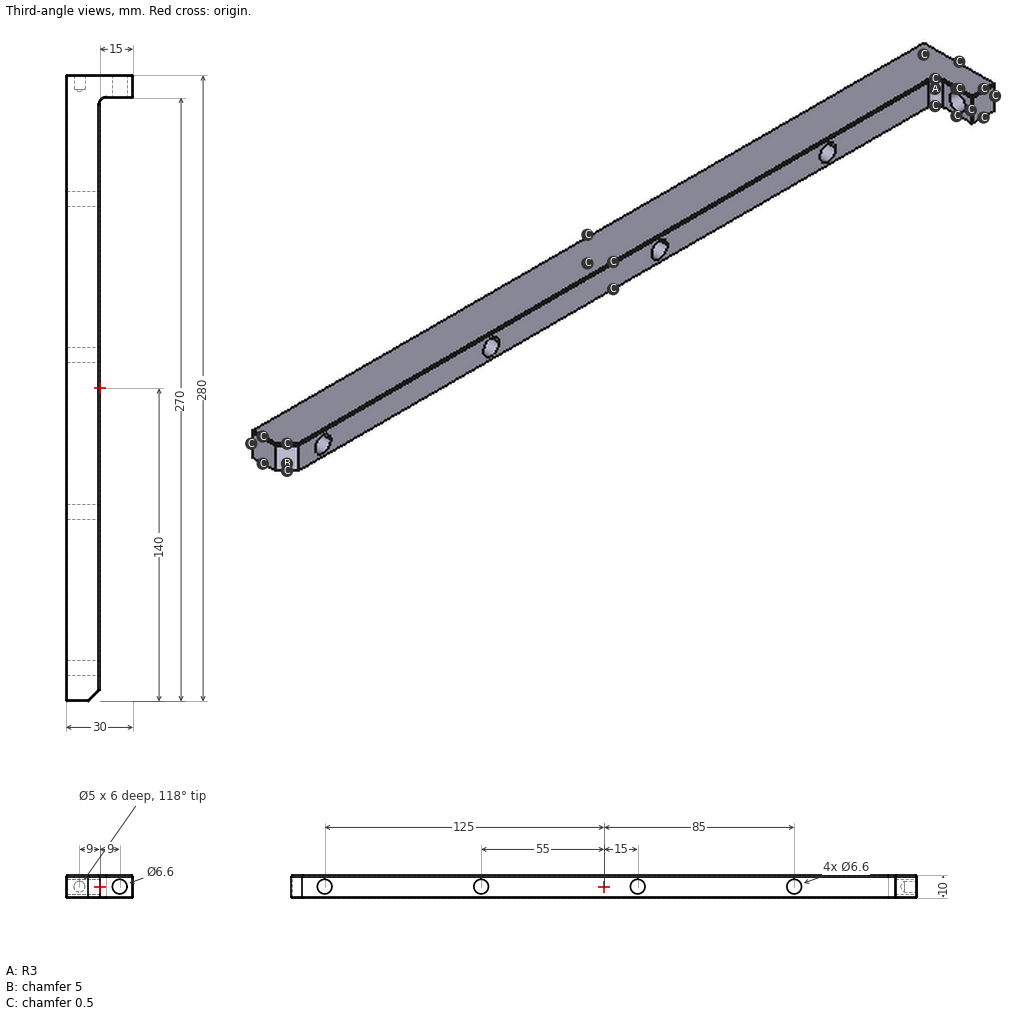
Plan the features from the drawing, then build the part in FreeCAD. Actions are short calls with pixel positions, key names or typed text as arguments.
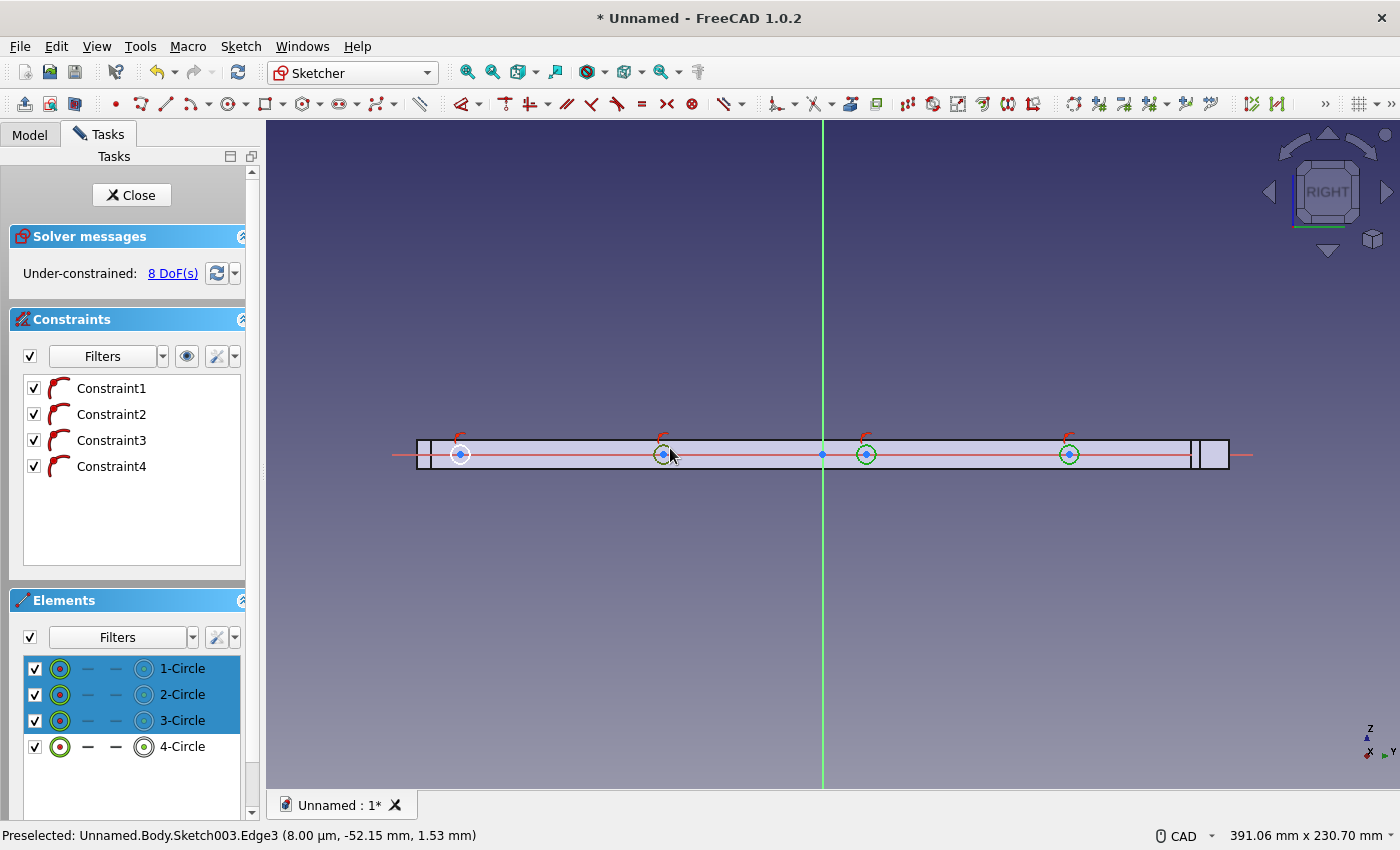
scroll(467, 448, up, 4)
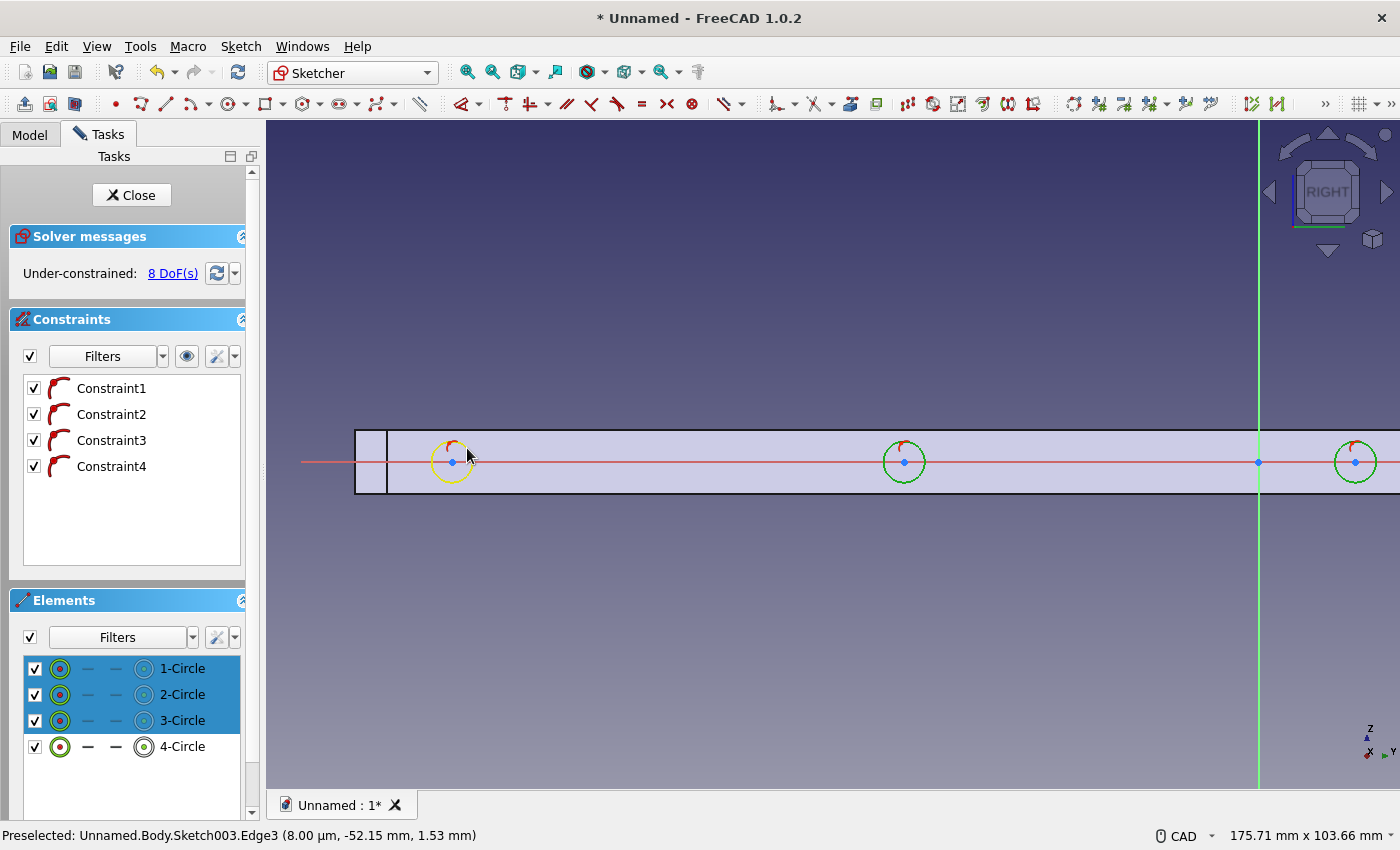
click(467, 447)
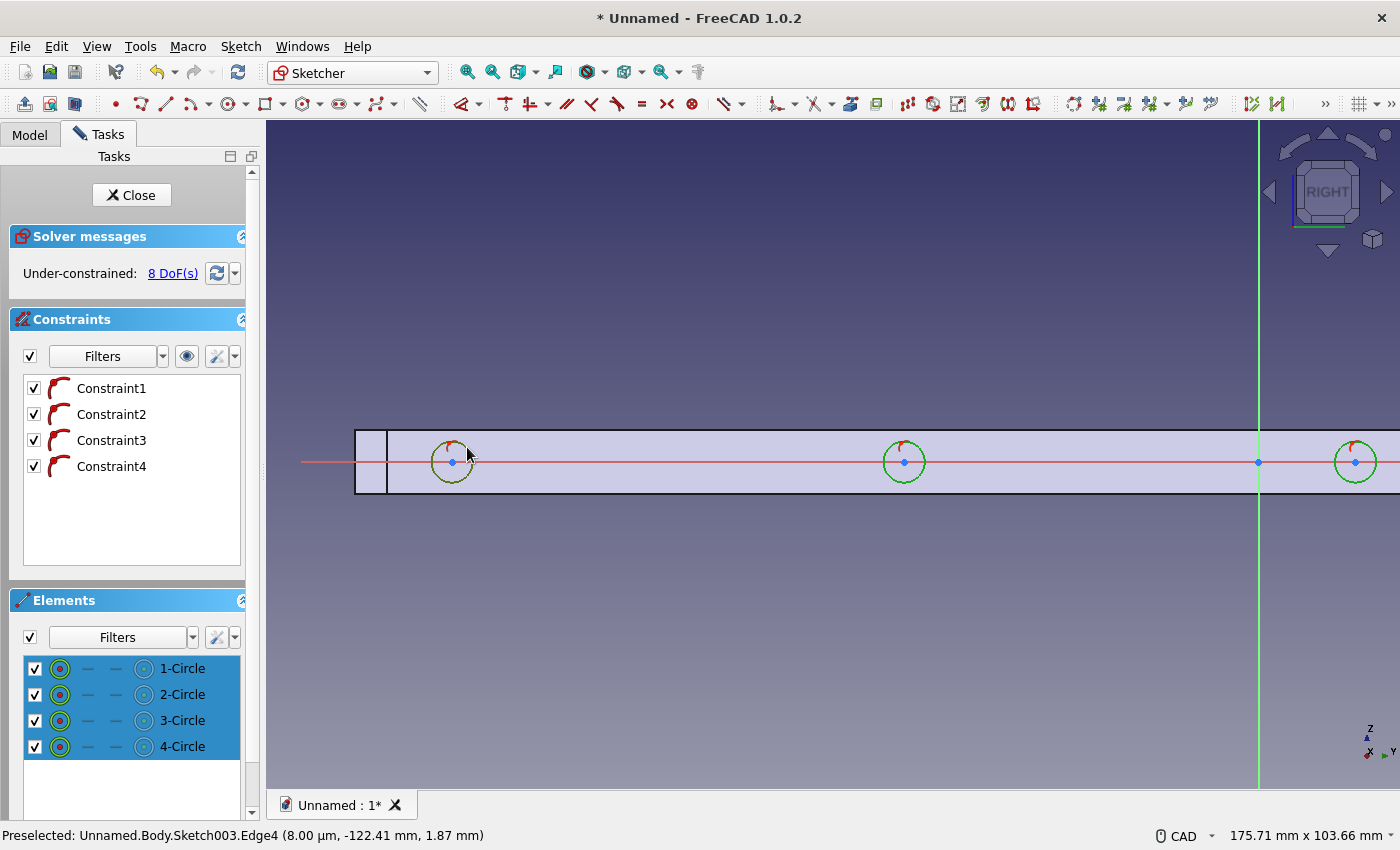
key(e)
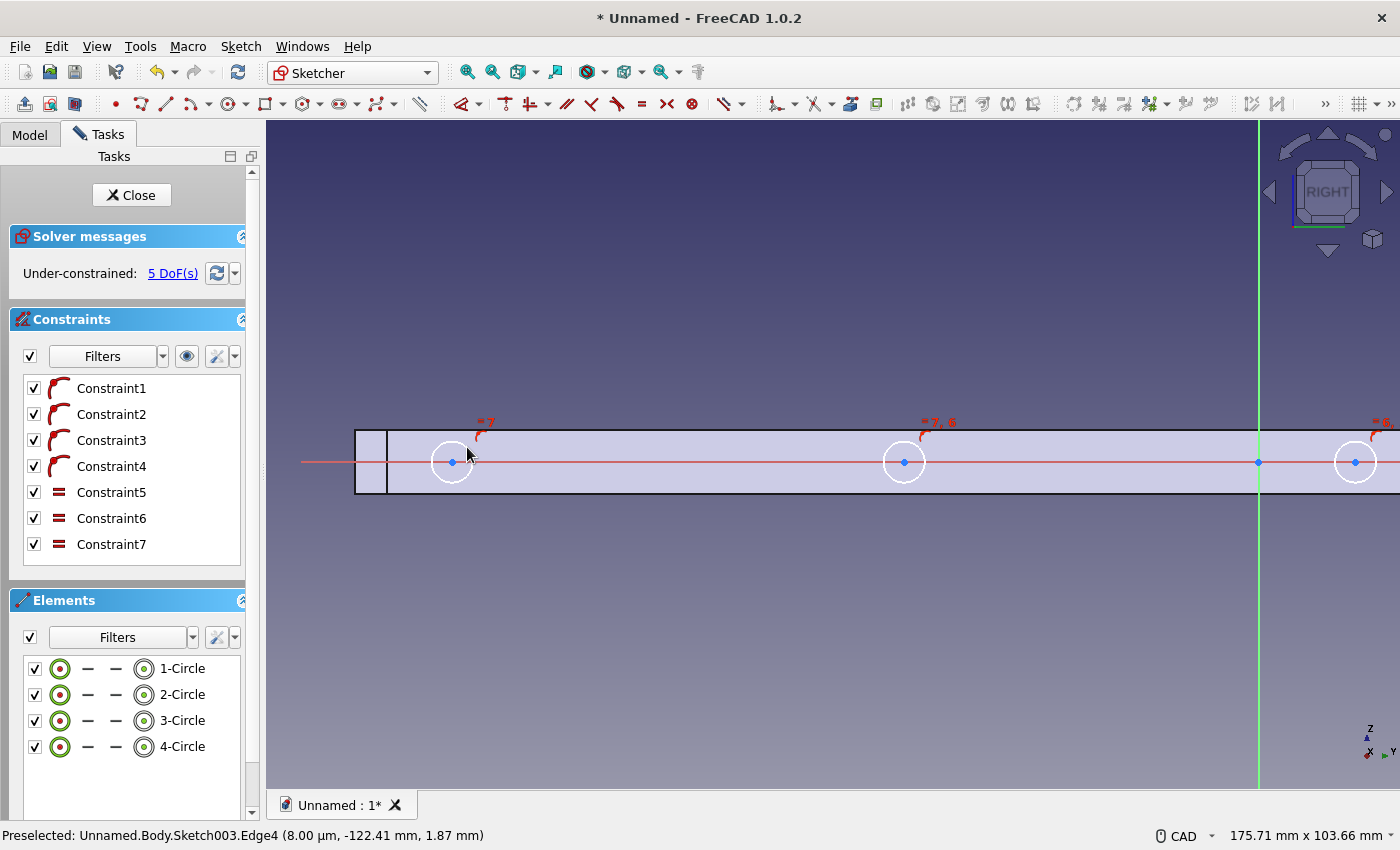
key(d)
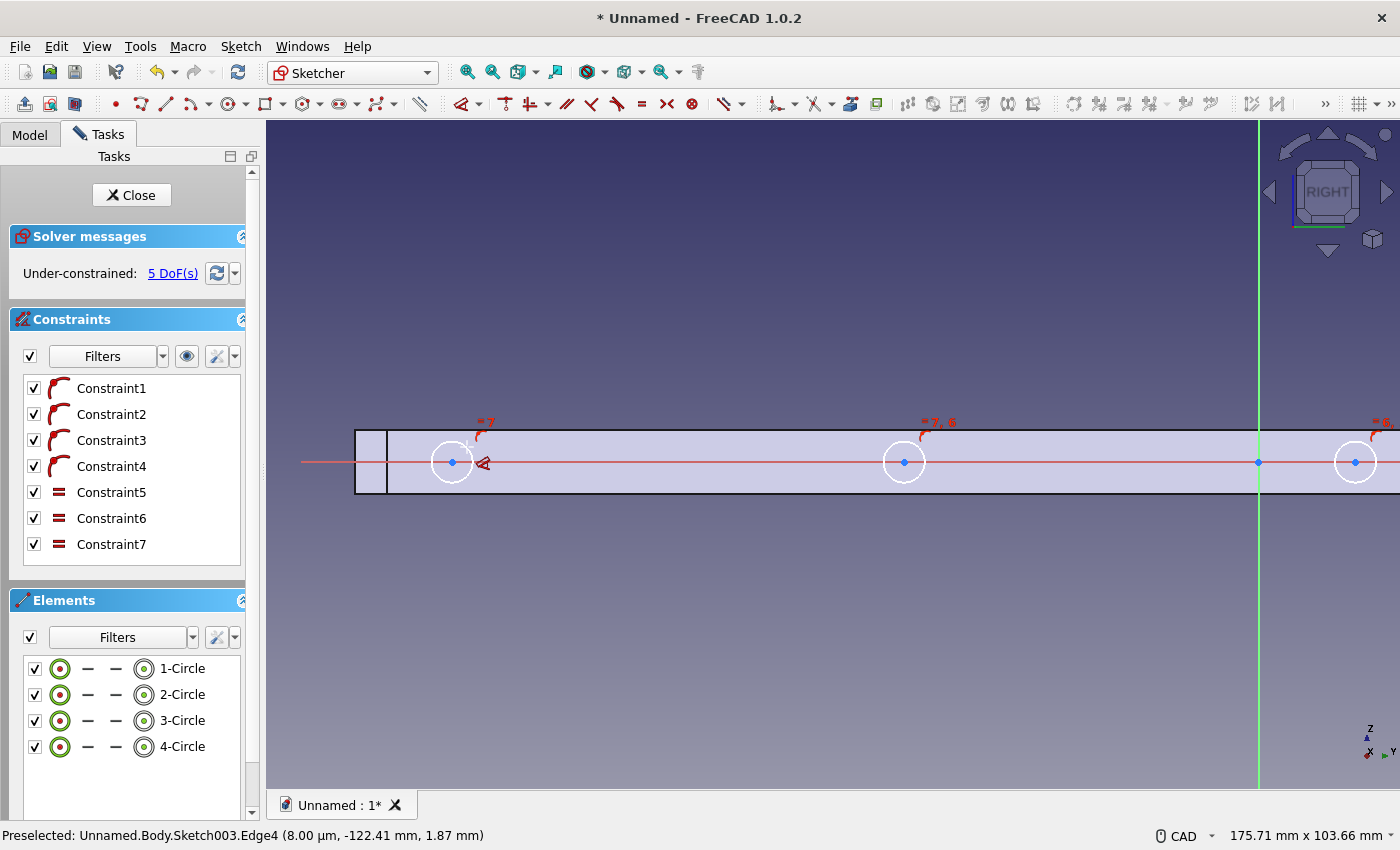
scroll(467, 448, down, 4)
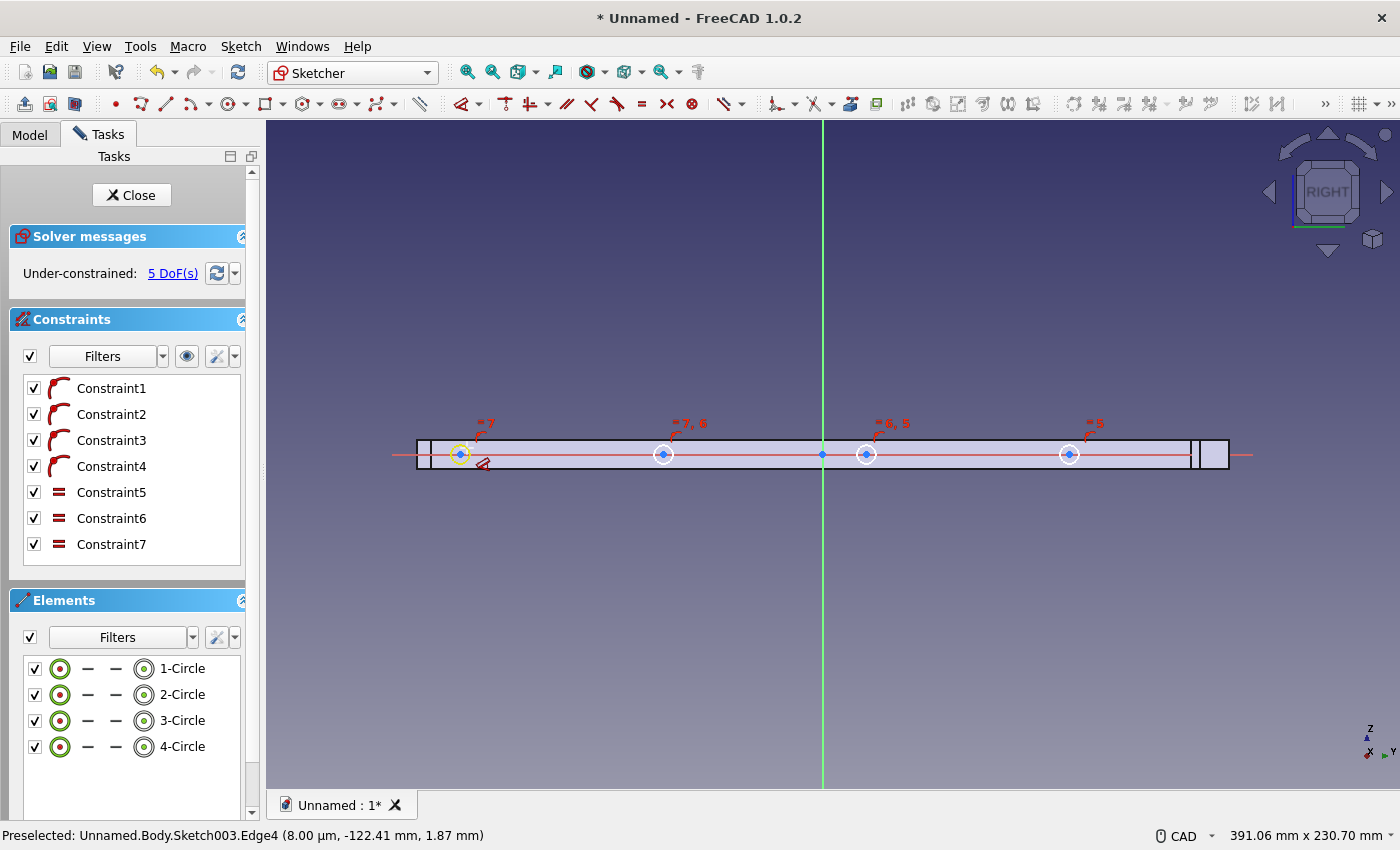
scroll(1076, 448, up, 4)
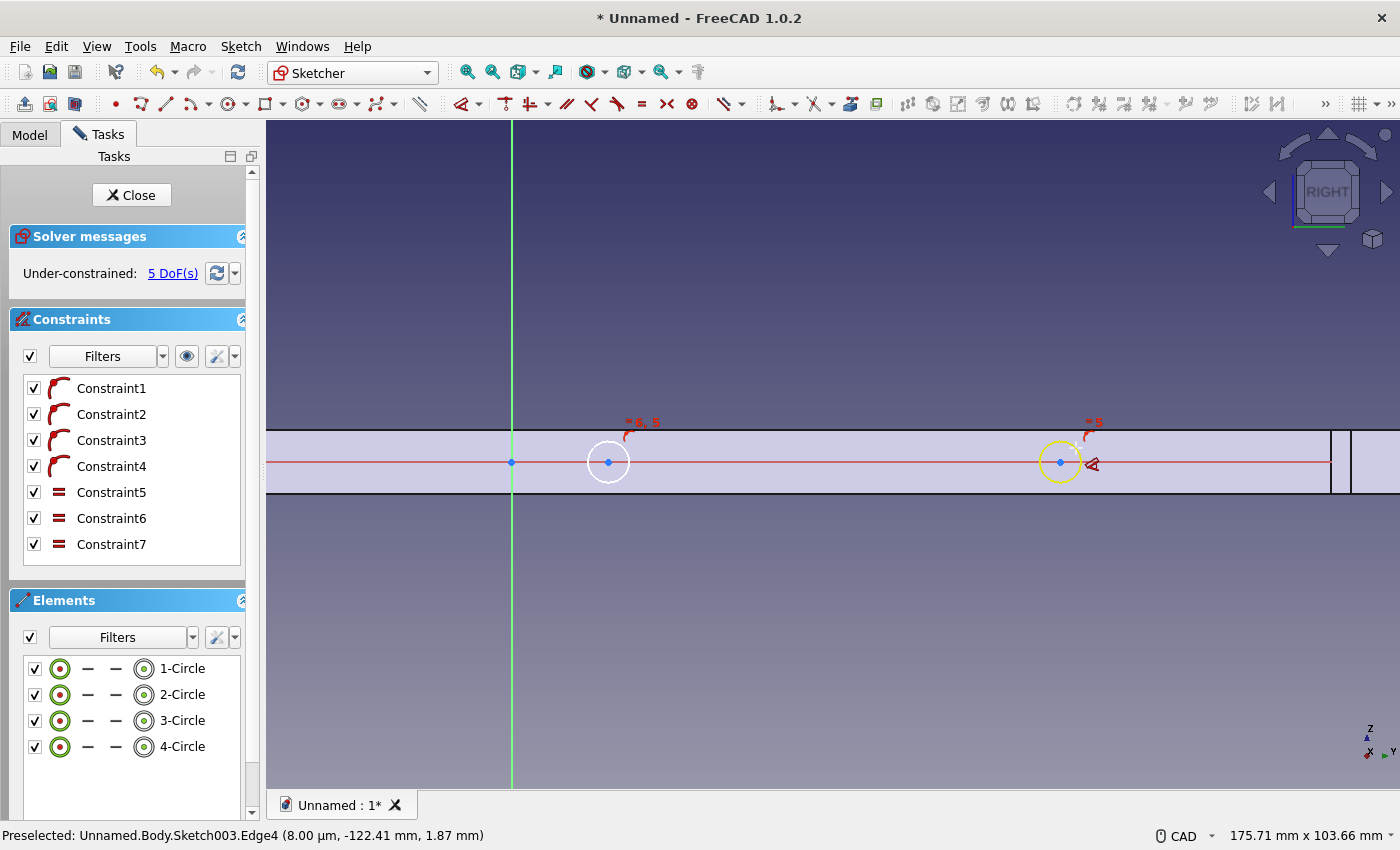
click(1075, 447)
click(1097, 424)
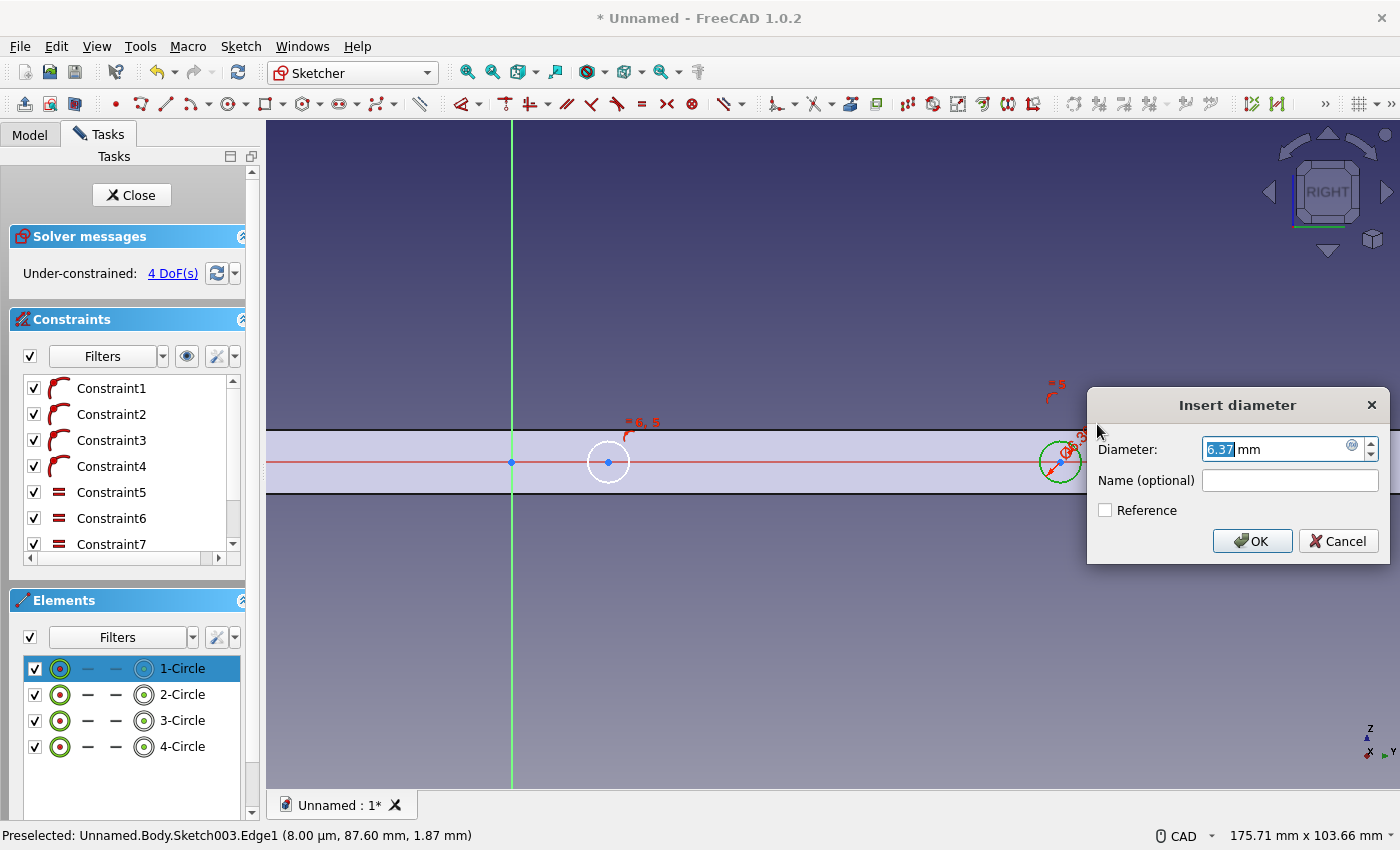
text(6.6)
key(Return)